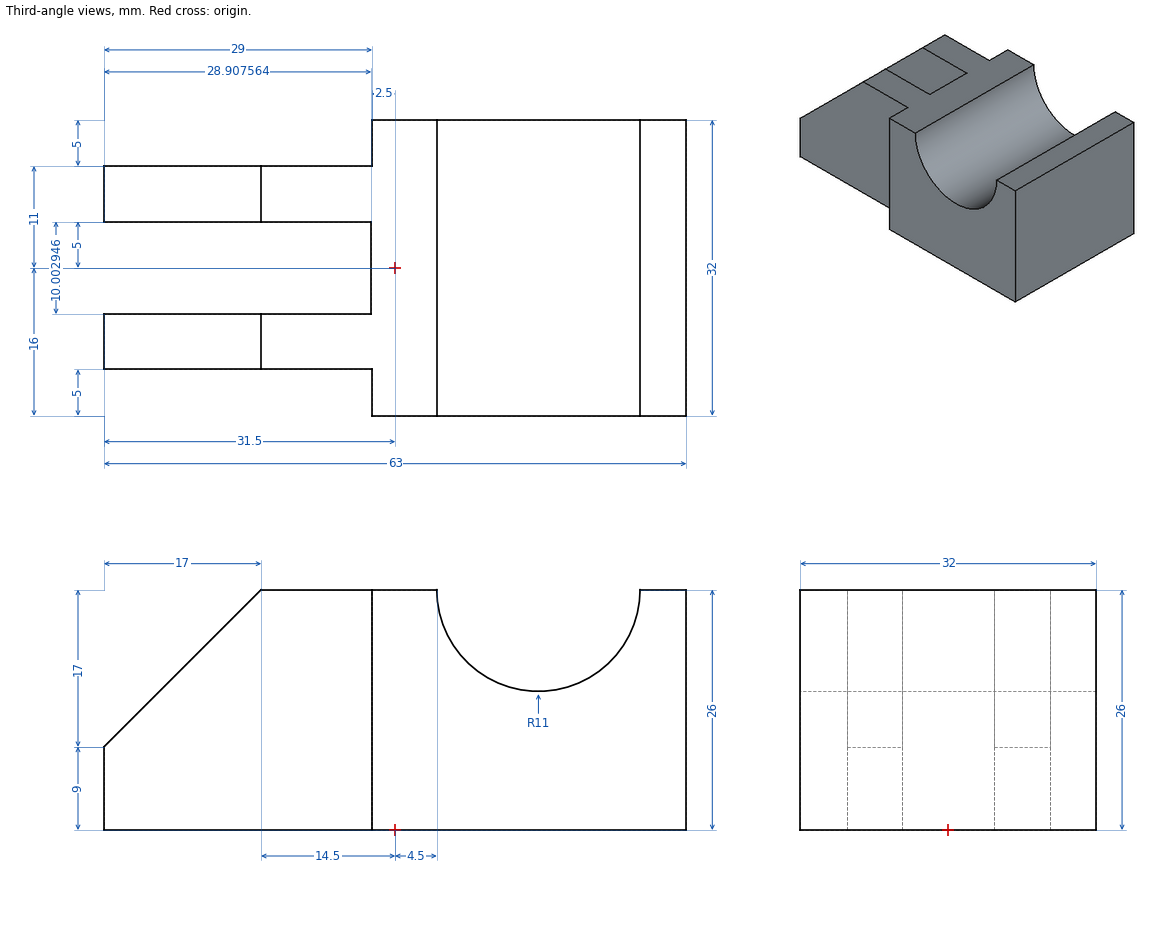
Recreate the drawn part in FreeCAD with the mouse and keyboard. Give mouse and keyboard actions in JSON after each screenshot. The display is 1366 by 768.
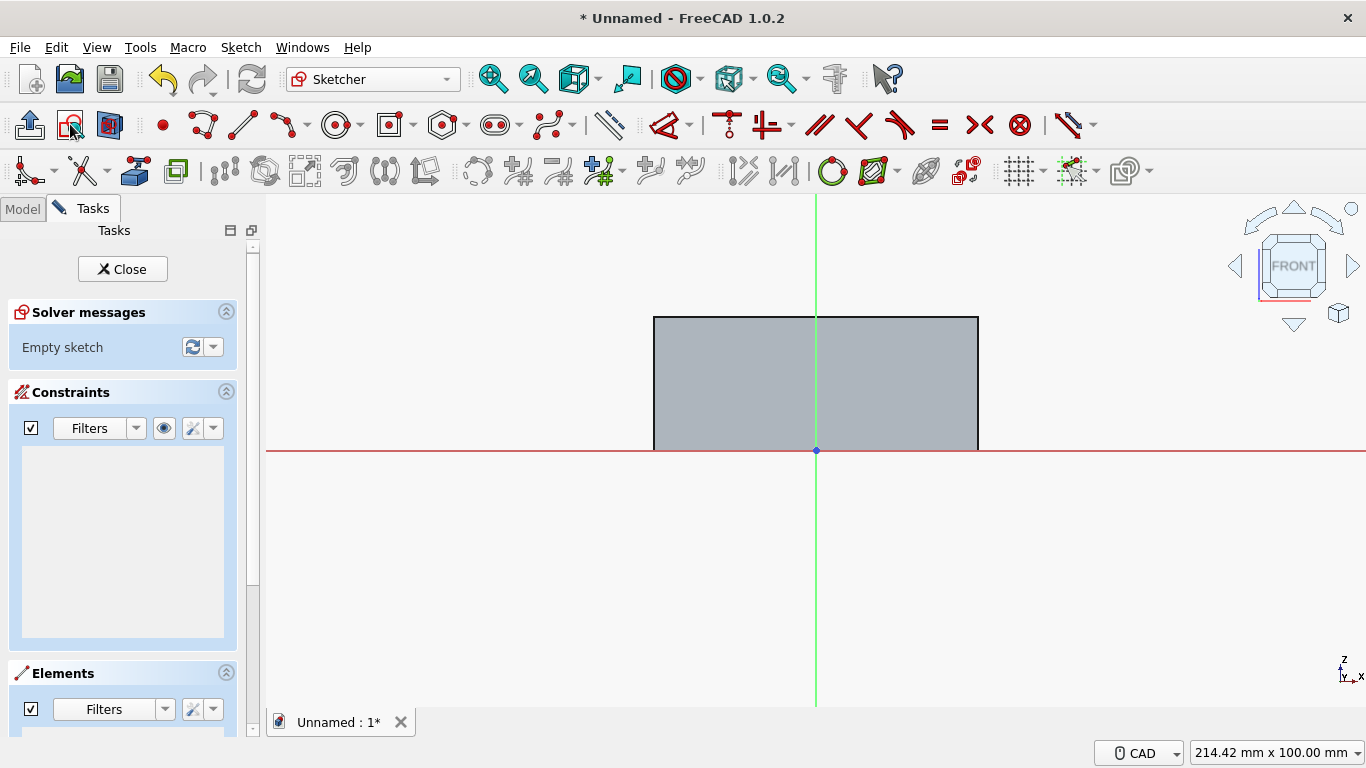
{"action": "scroll", "coordinate": [995, 329], "scroll_direction": "up", "scroll_amount": 4}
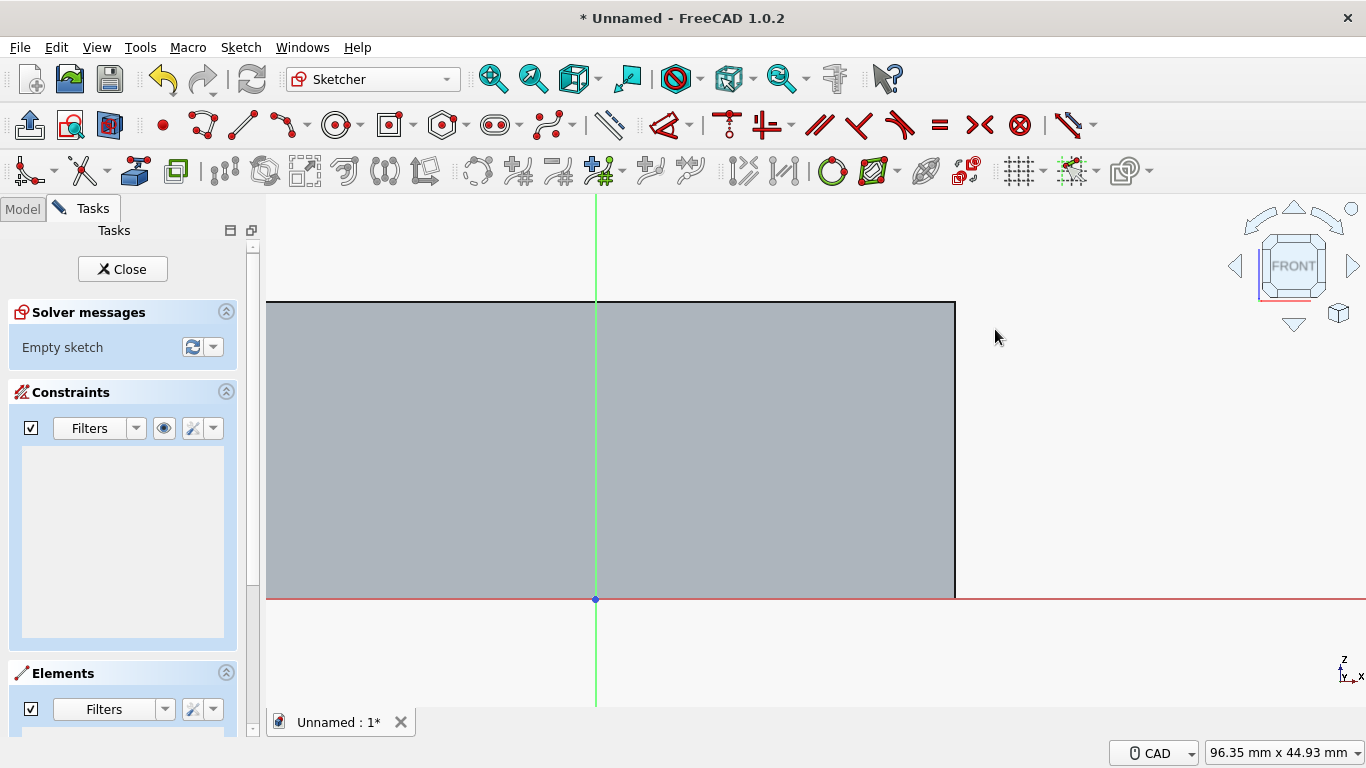
{"action": "left_click", "coordinate": [244, 126]}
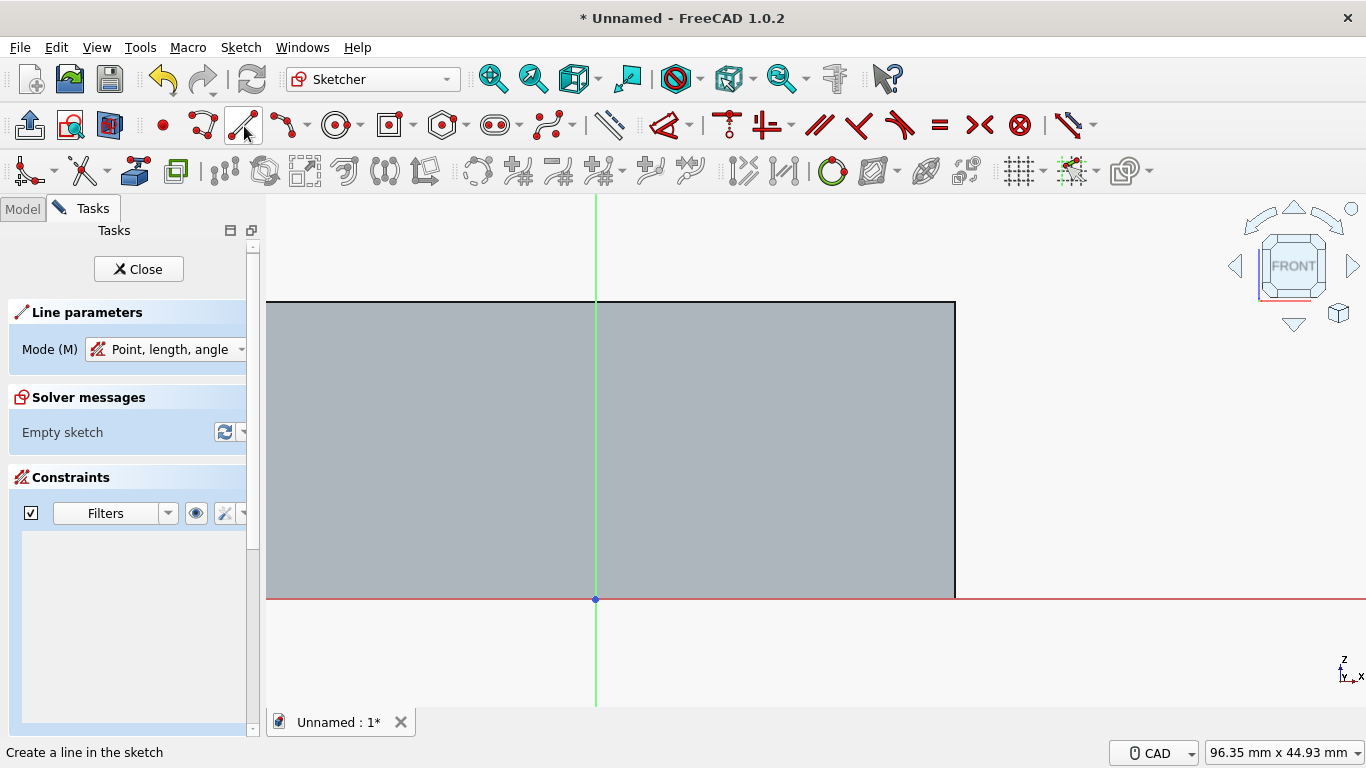
{"action": "left_click", "coordinate": [898, 302]}
{"action": "left_click", "coordinate": [647, 302]}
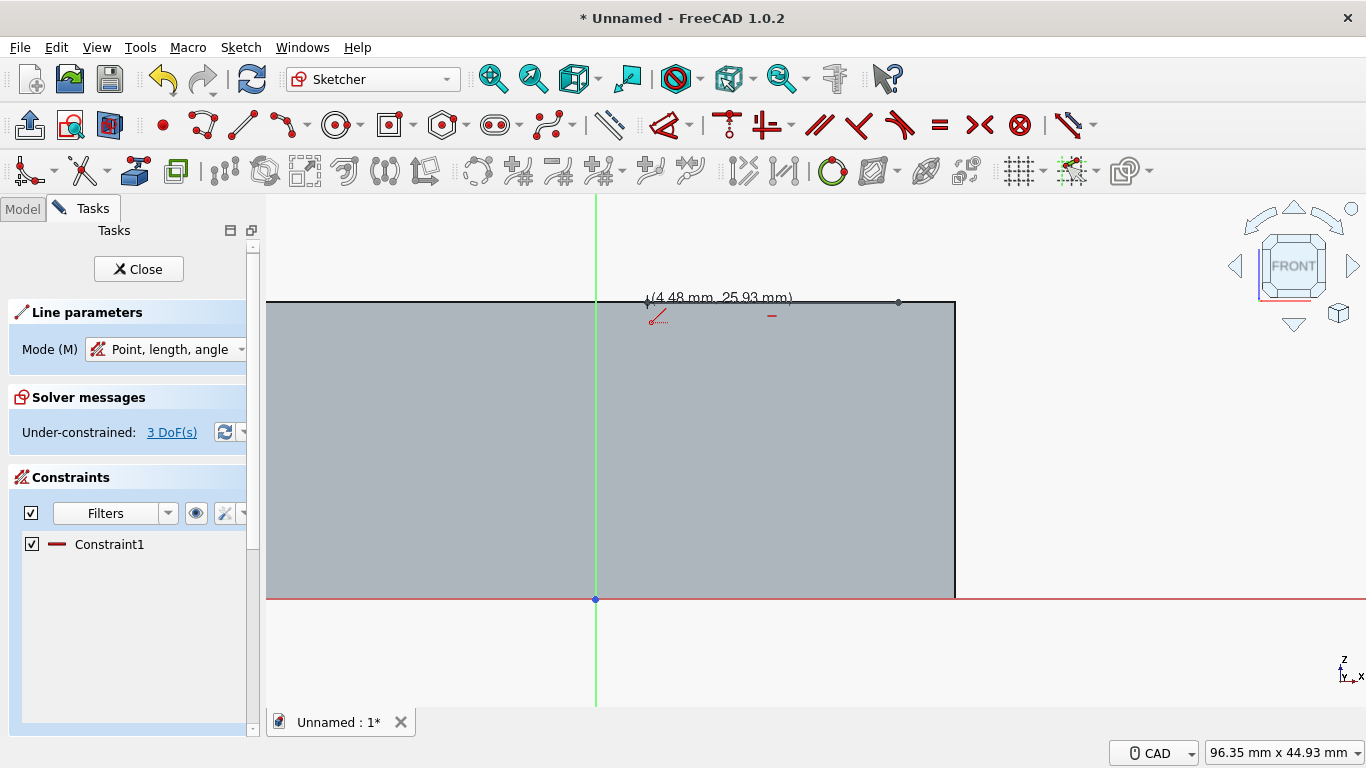
{"action": "left_click", "coordinate": [284, 126]}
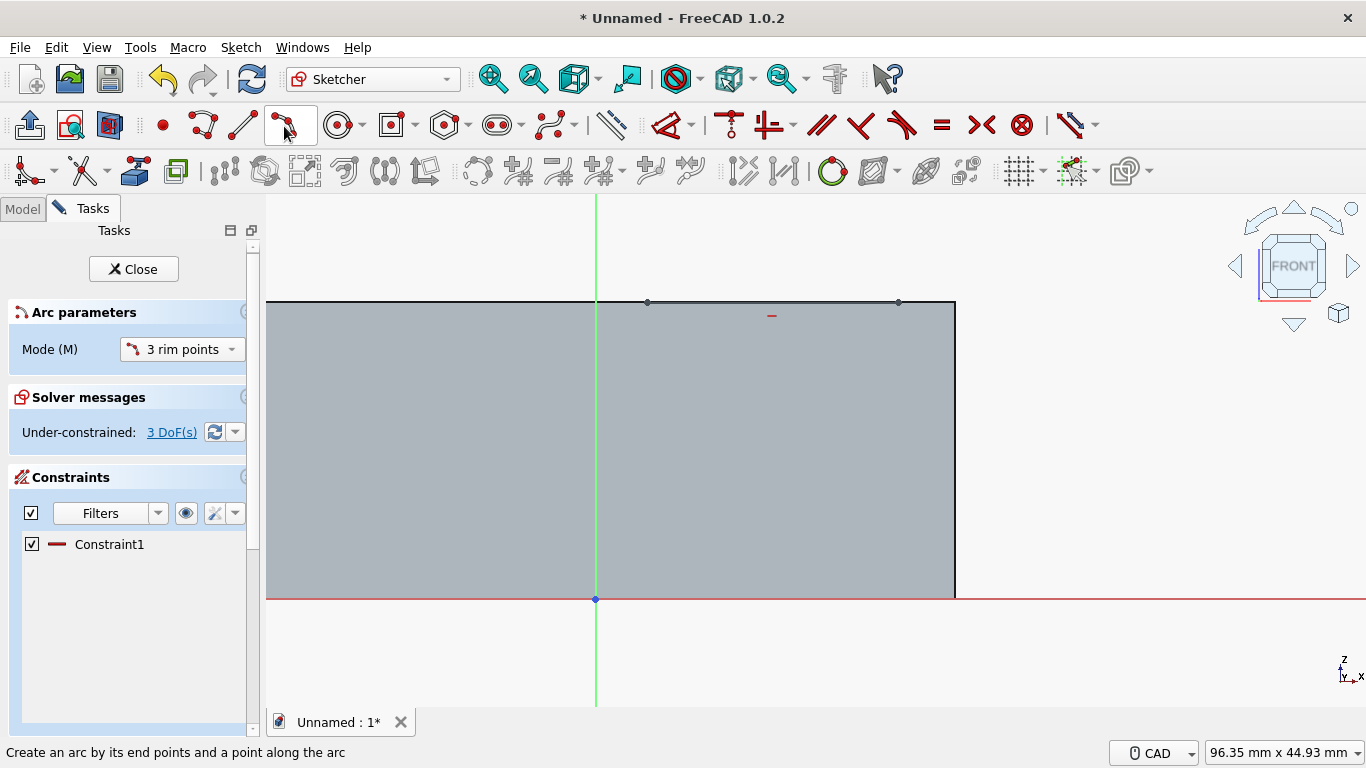
{"action": "left_click", "coordinate": [647, 303]}
{"action": "left_click", "coordinate": [898, 303]}
{"action": "left_click", "coordinate": [773, 428]}
{"action": "key", "text": "Escape"}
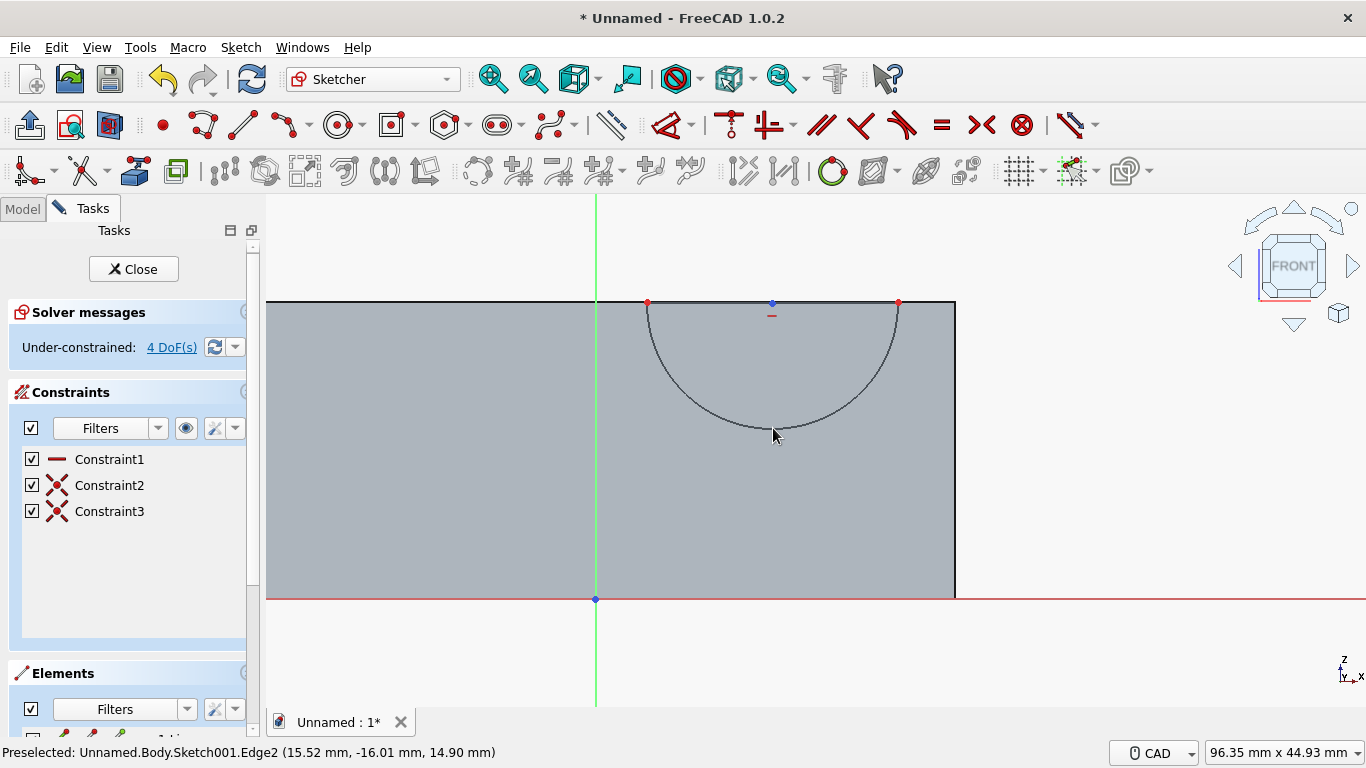
{"action": "left_click", "coordinate": [666, 126]}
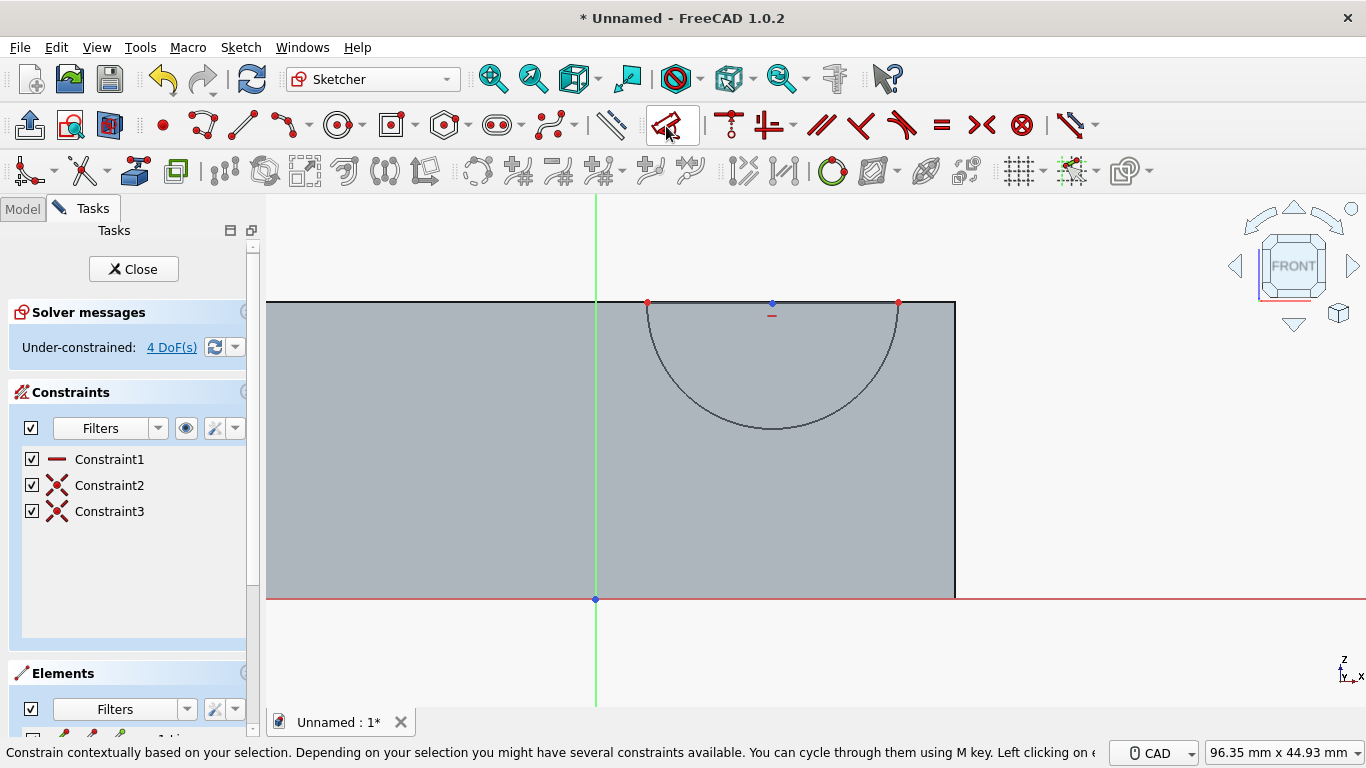
{"action": "left_click", "coordinate": [699, 405]}
{"action": "left_click", "coordinate": [680, 431]}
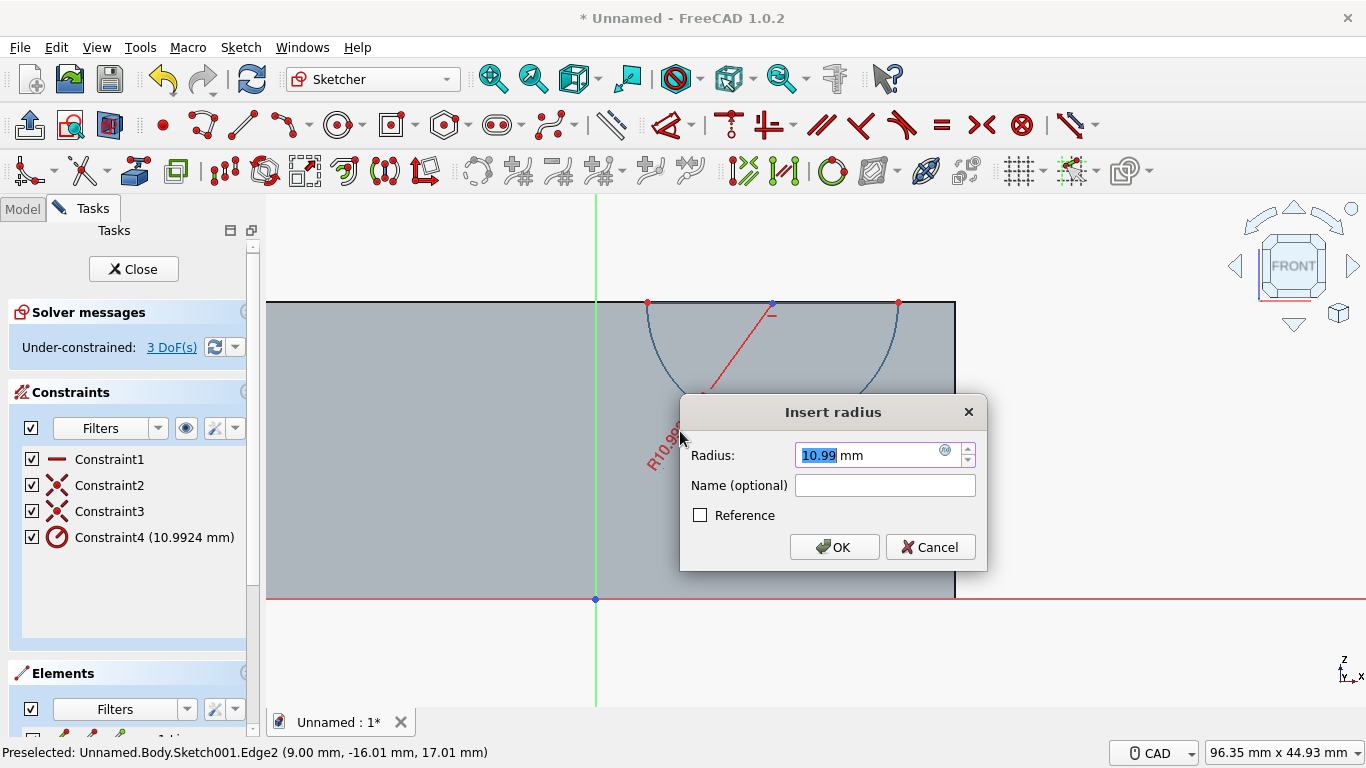
{"action": "type", "text": "11"}
{"action": "key", "text": "Return"}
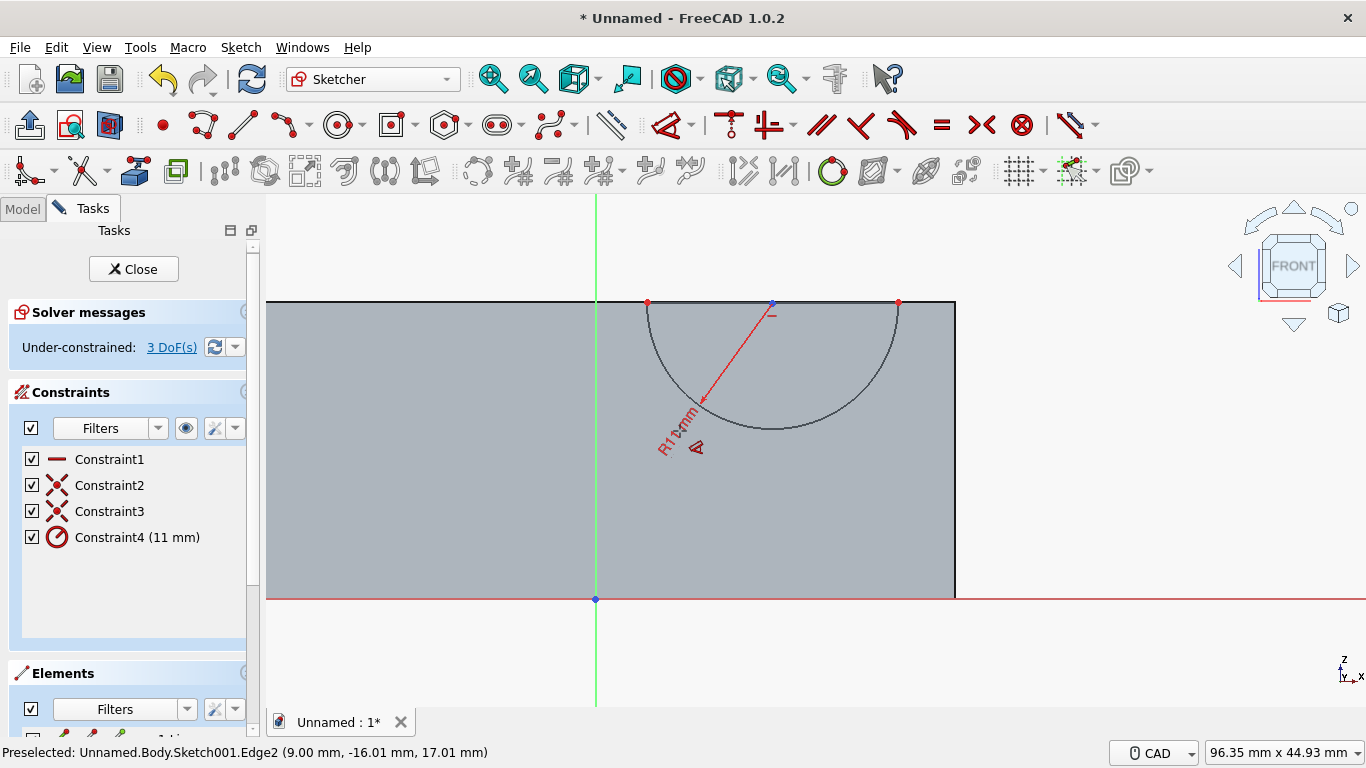
{"action": "left_click", "coordinate": [898, 303]}
{"action": "left_click", "coordinate": [562, 451]}